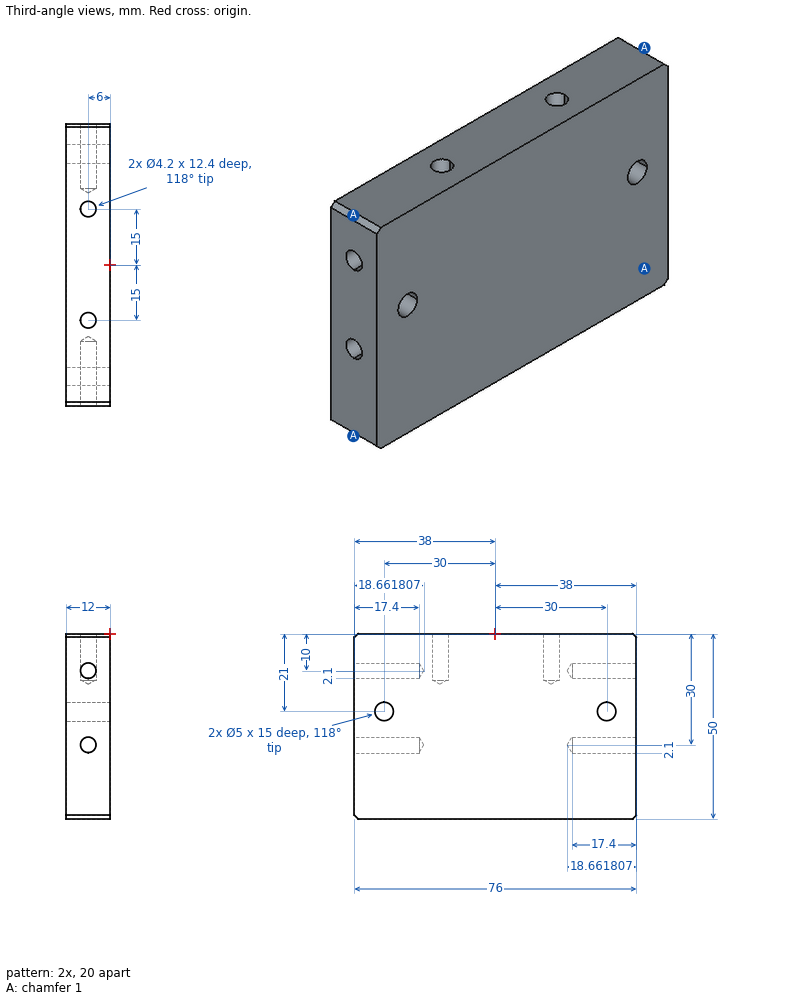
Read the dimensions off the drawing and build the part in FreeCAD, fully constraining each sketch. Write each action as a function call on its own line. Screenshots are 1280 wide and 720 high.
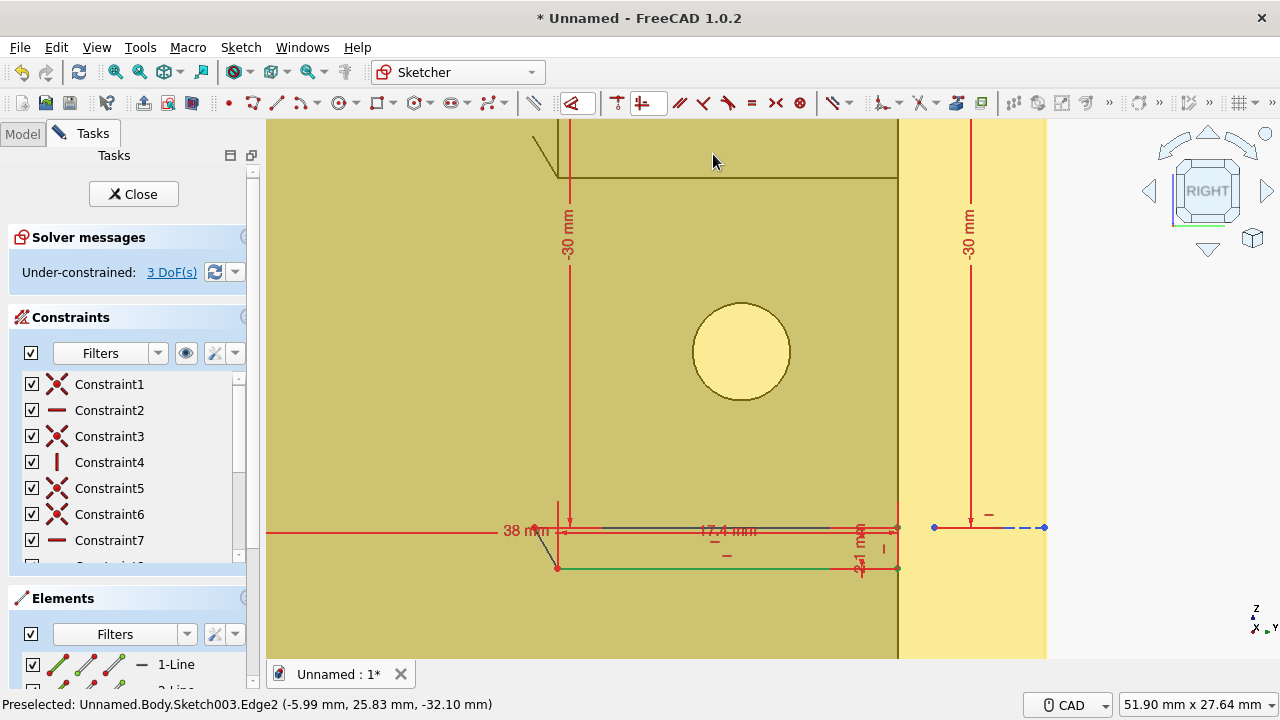
click(789, 528)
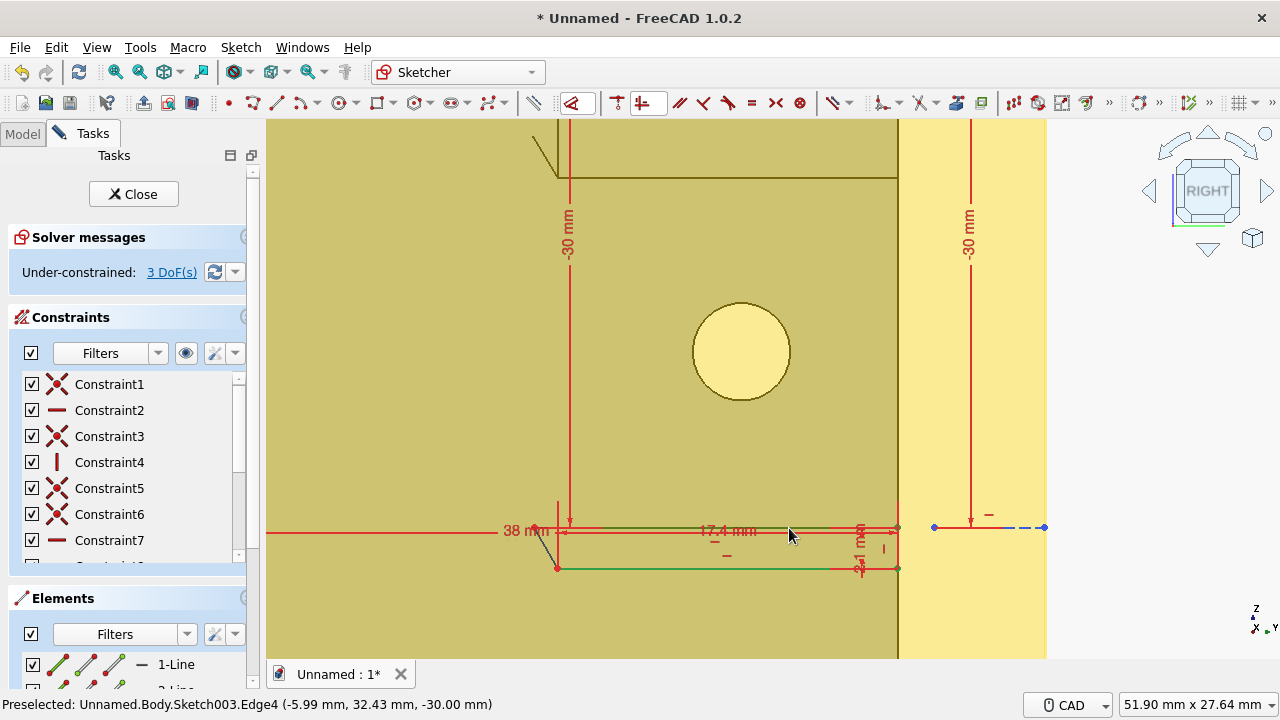
click(590, 104)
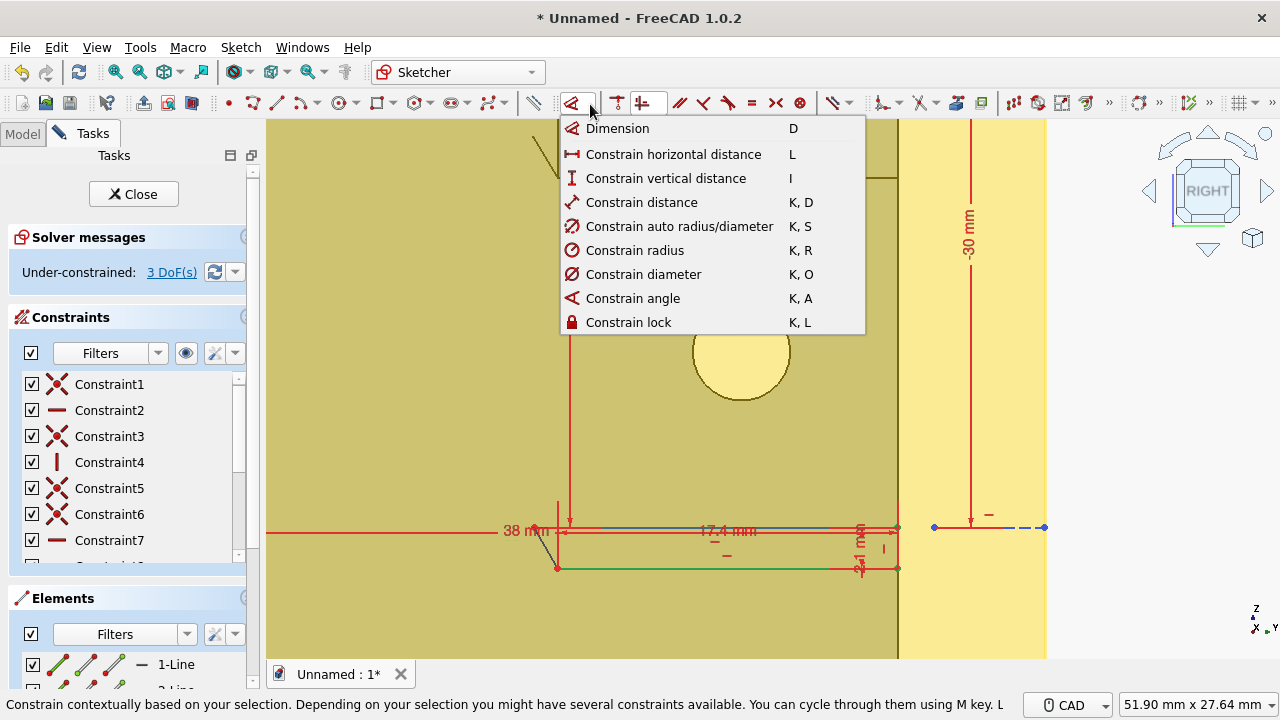
click(713, 154)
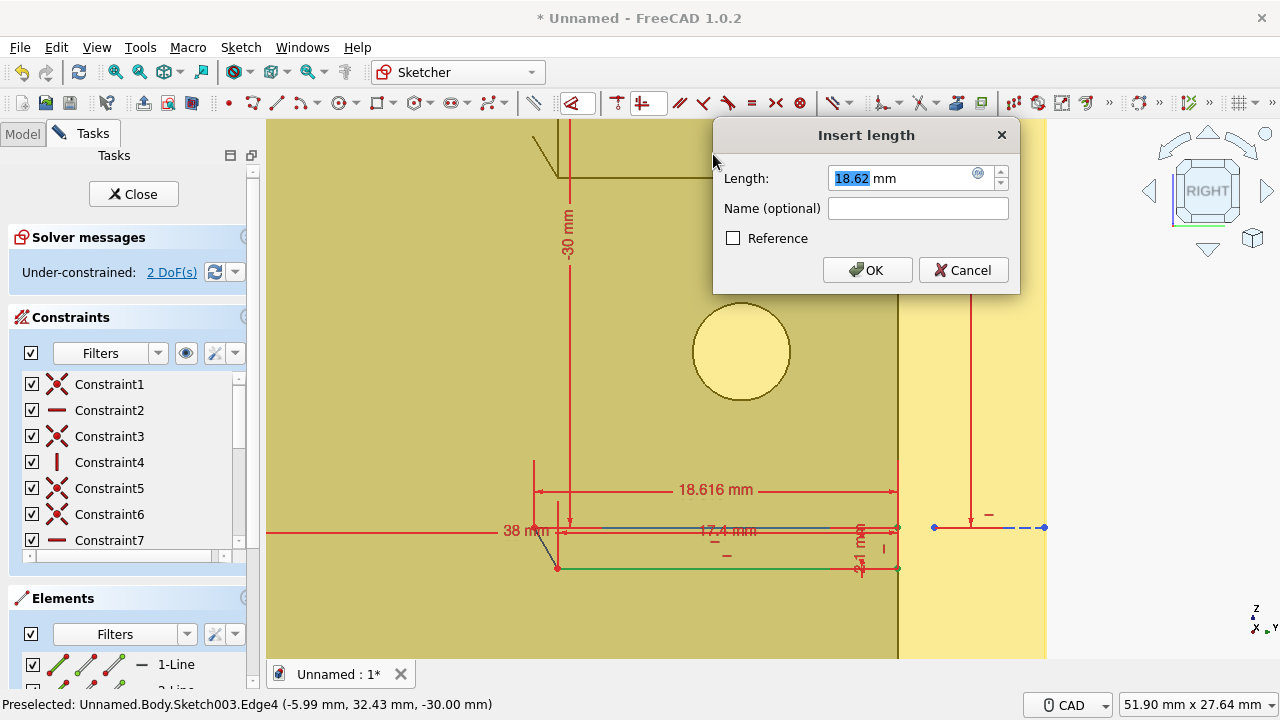
text(18.661807)
key(Return)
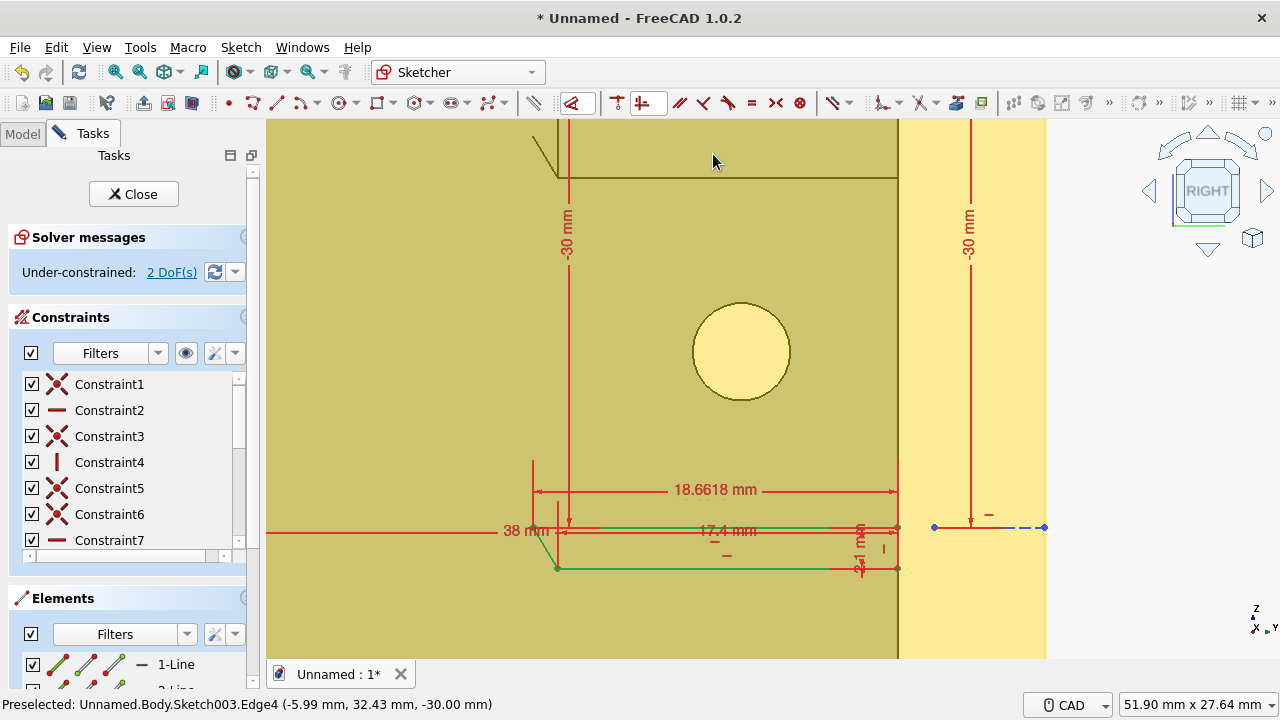
click(134, 194)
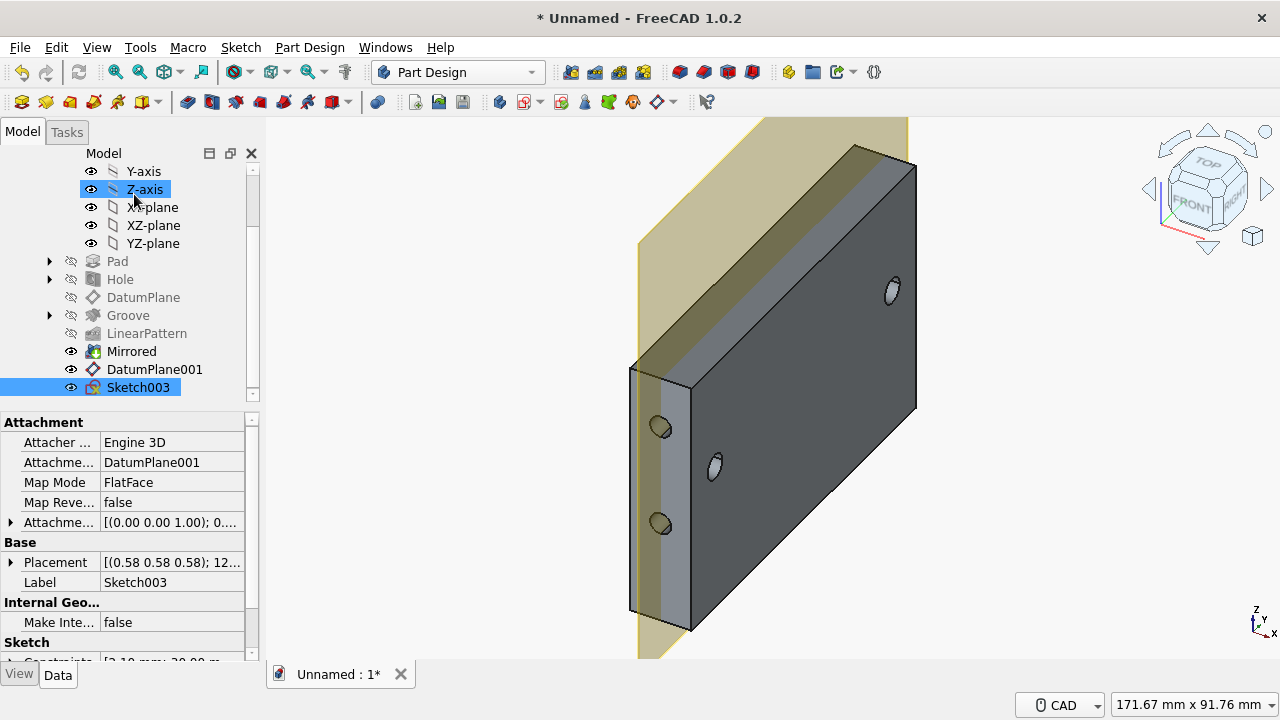
click(236, 102)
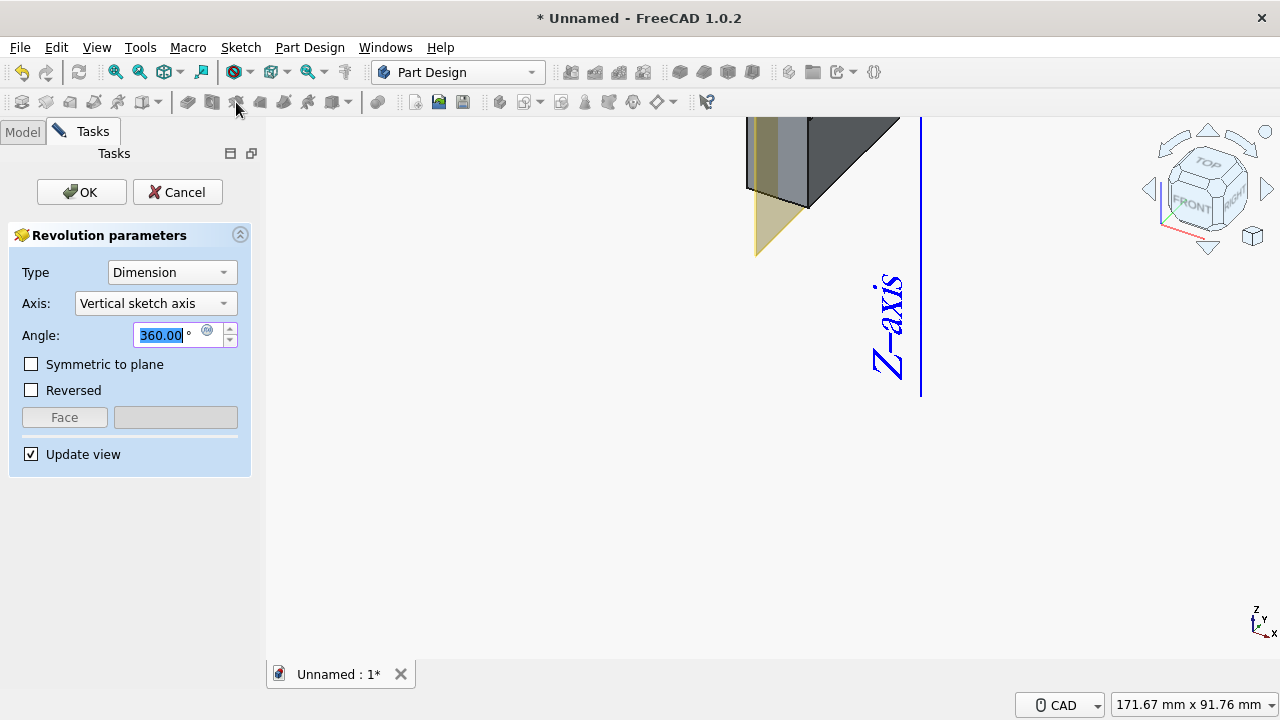
click(156, 304)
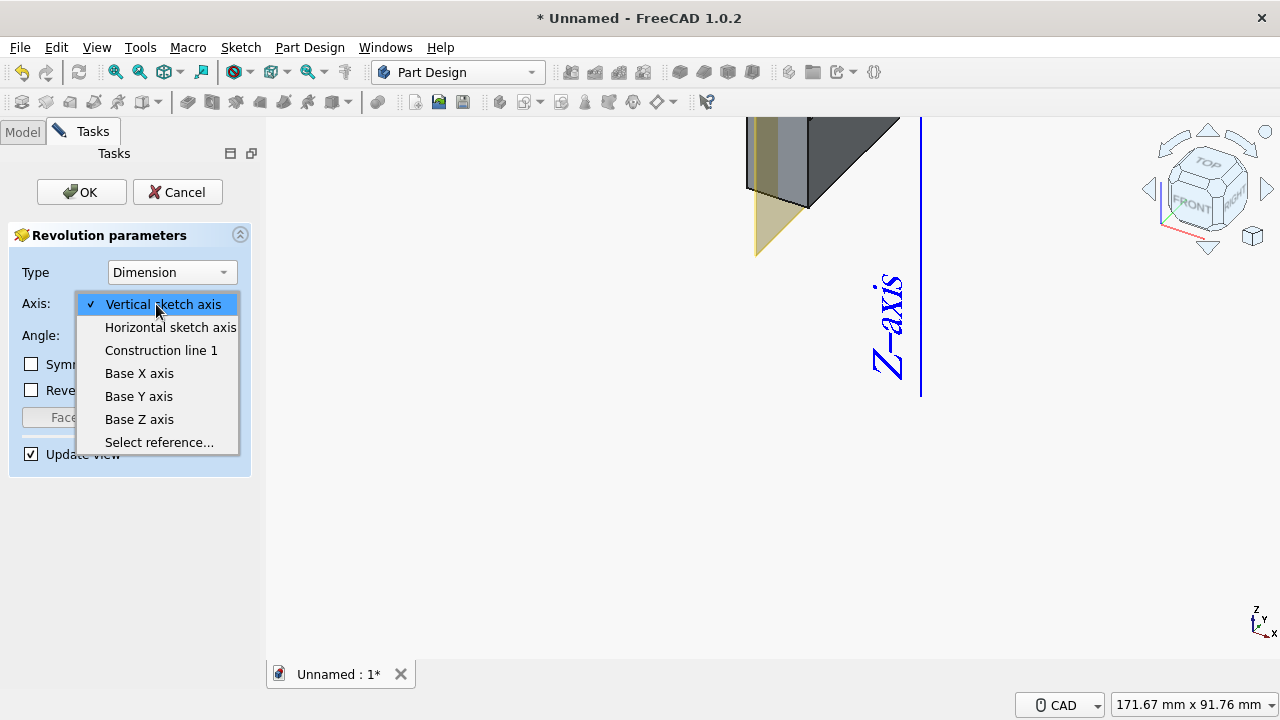
click(156, 350)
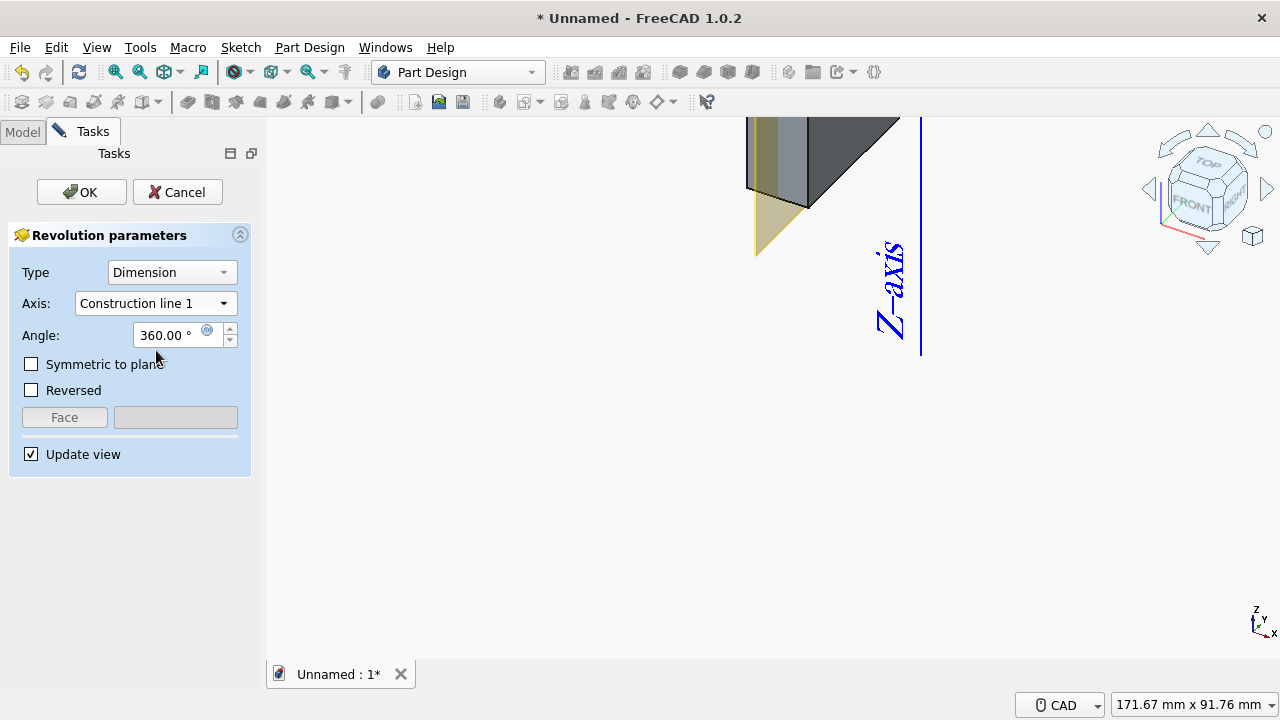
click(82, 192)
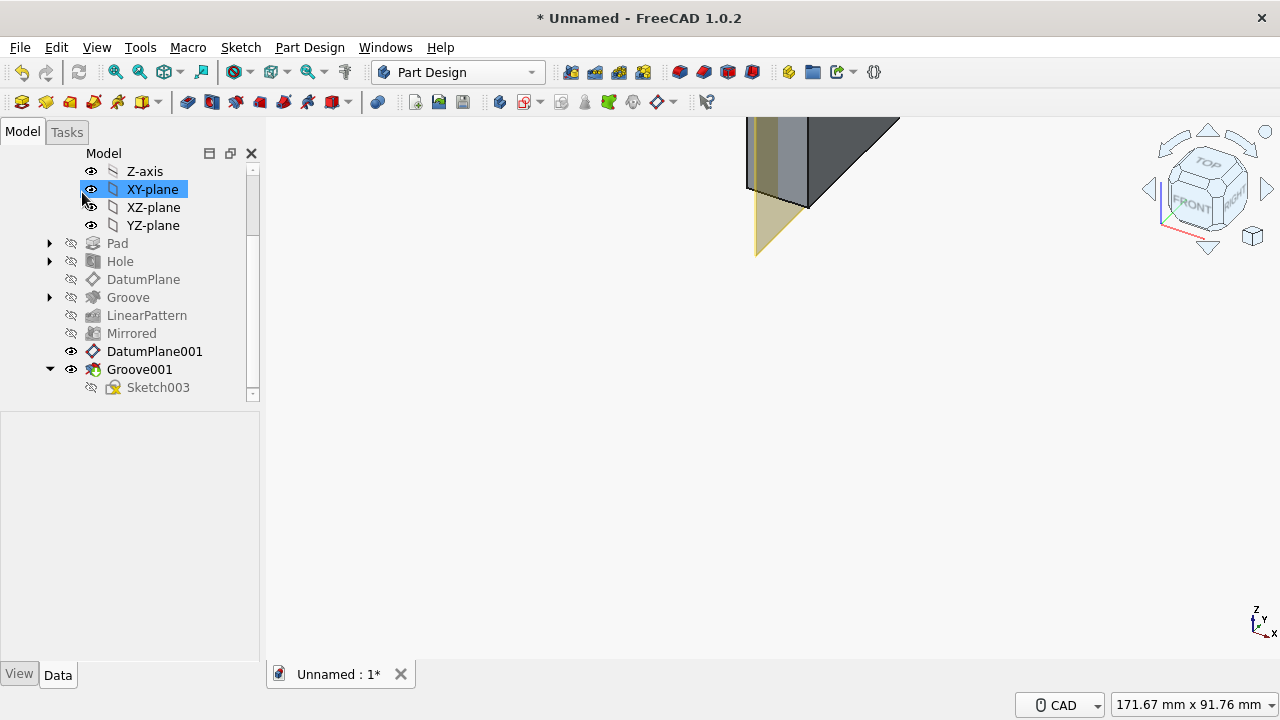
click(116, 351)
key(space)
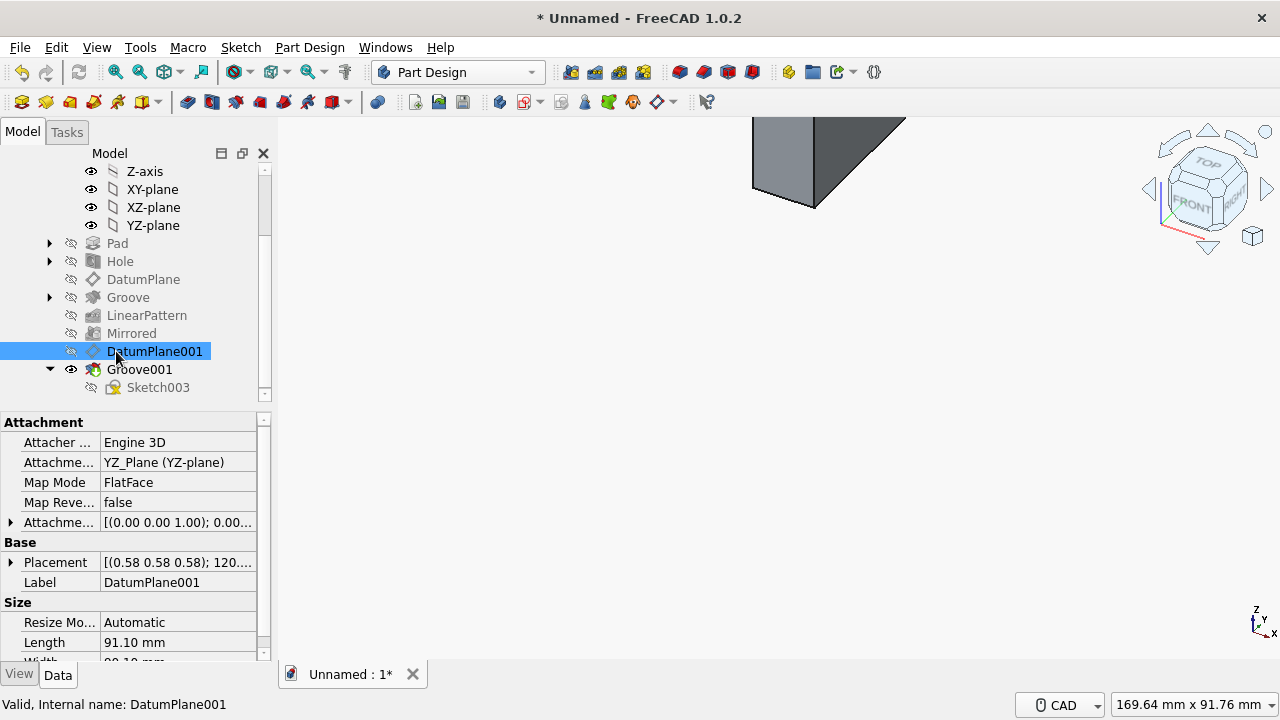
click(116, 72)